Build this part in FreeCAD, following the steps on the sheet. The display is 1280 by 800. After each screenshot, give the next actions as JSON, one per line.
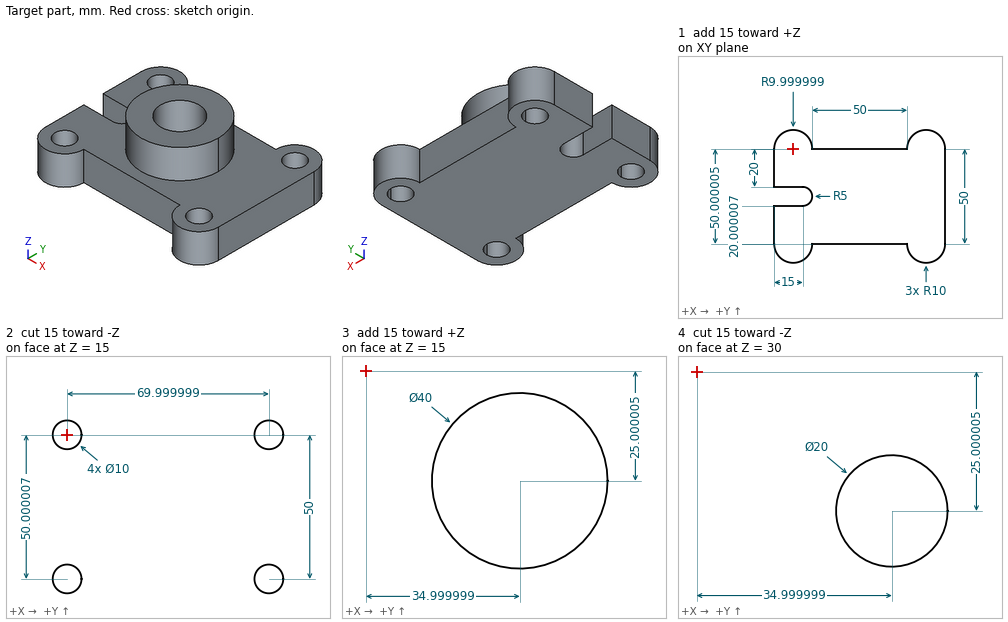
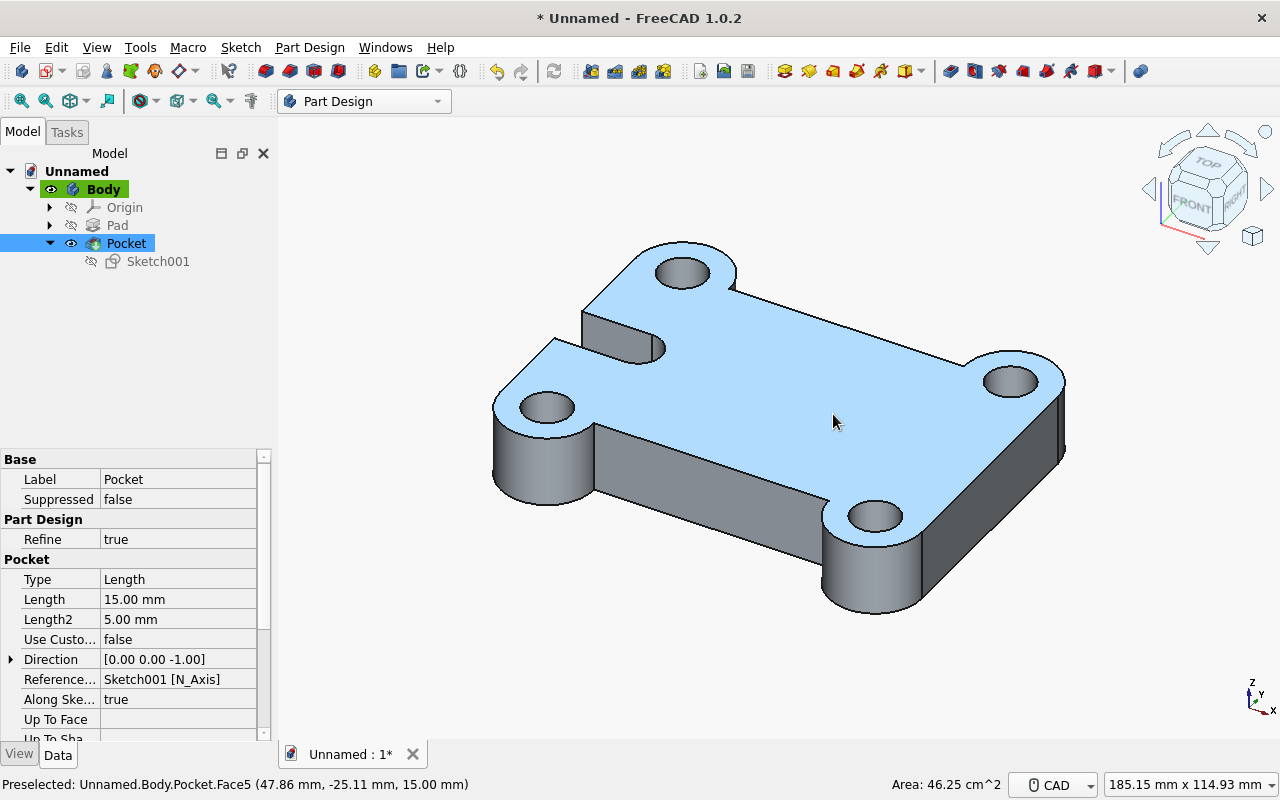
{"action": "left_click", "coordinate": [46, 72]}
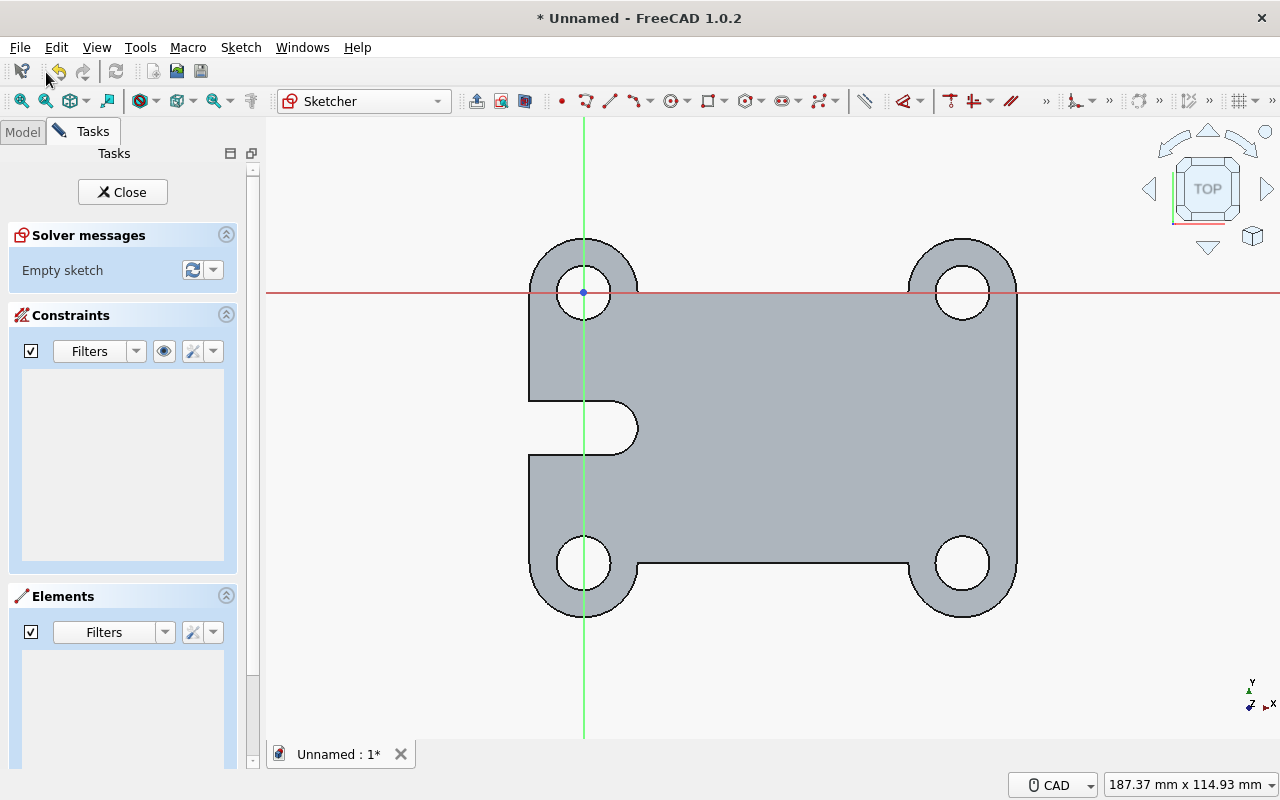
{"action": "scroll", "coordinate": [789, 387], "scroll_direction": "up", "scroll_amount": 2}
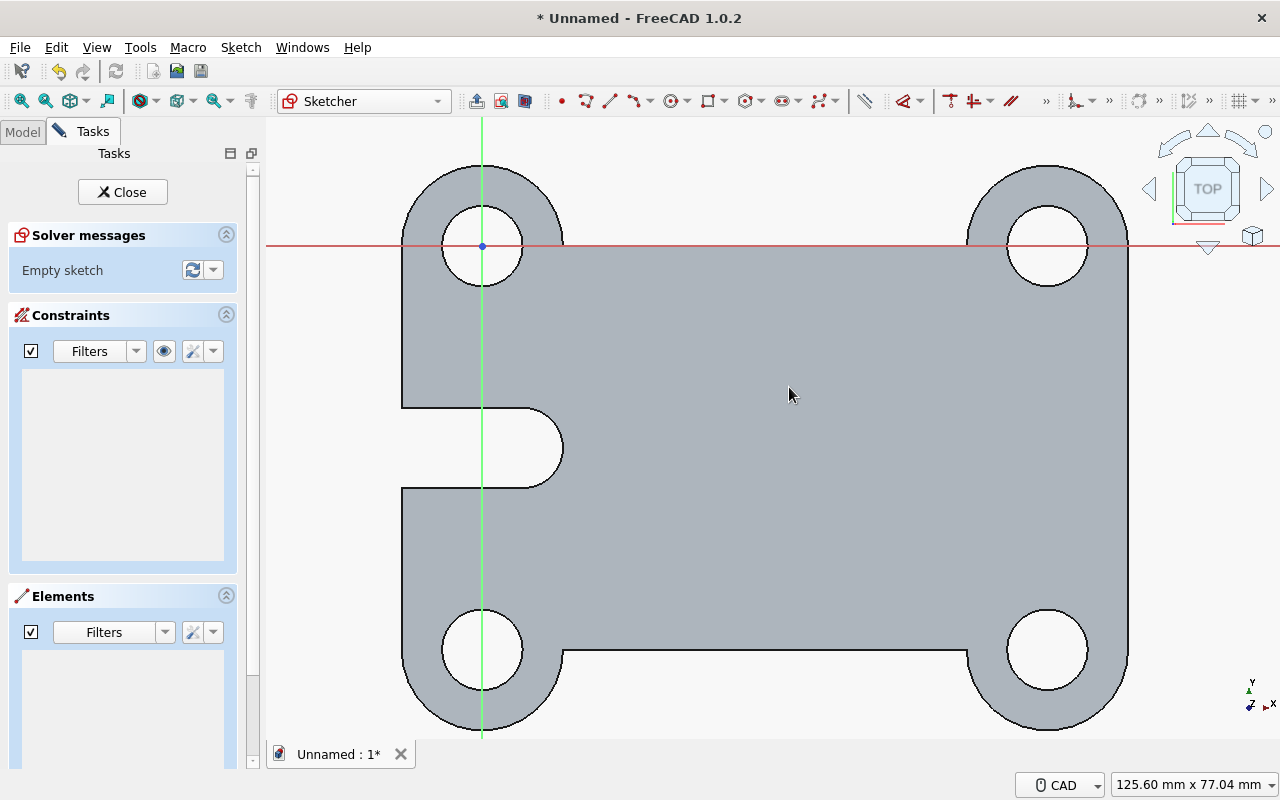
{"action": "left_click", "coordinate": [672, 102]}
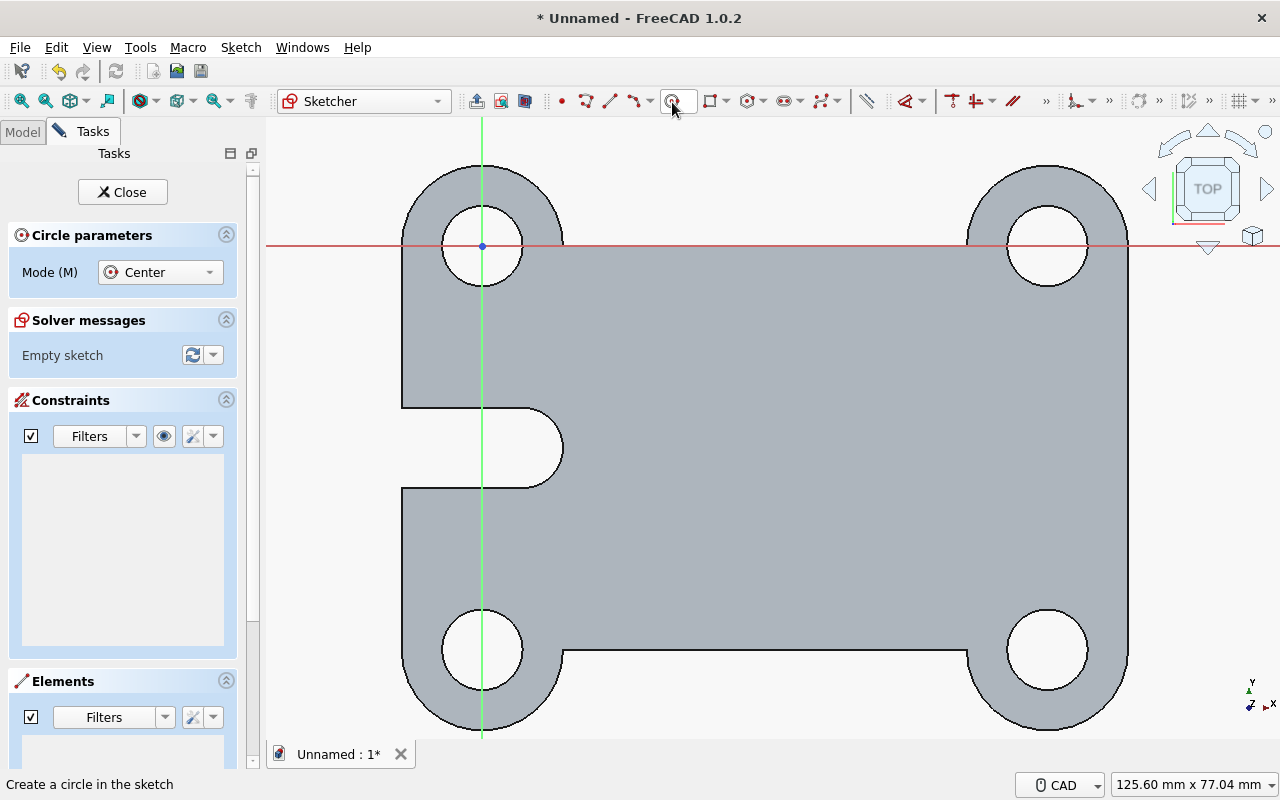
{"action": "left_click", "coordinate": [765, 448]}
{"action": "mouse_move", "coordinate": [879, 334]}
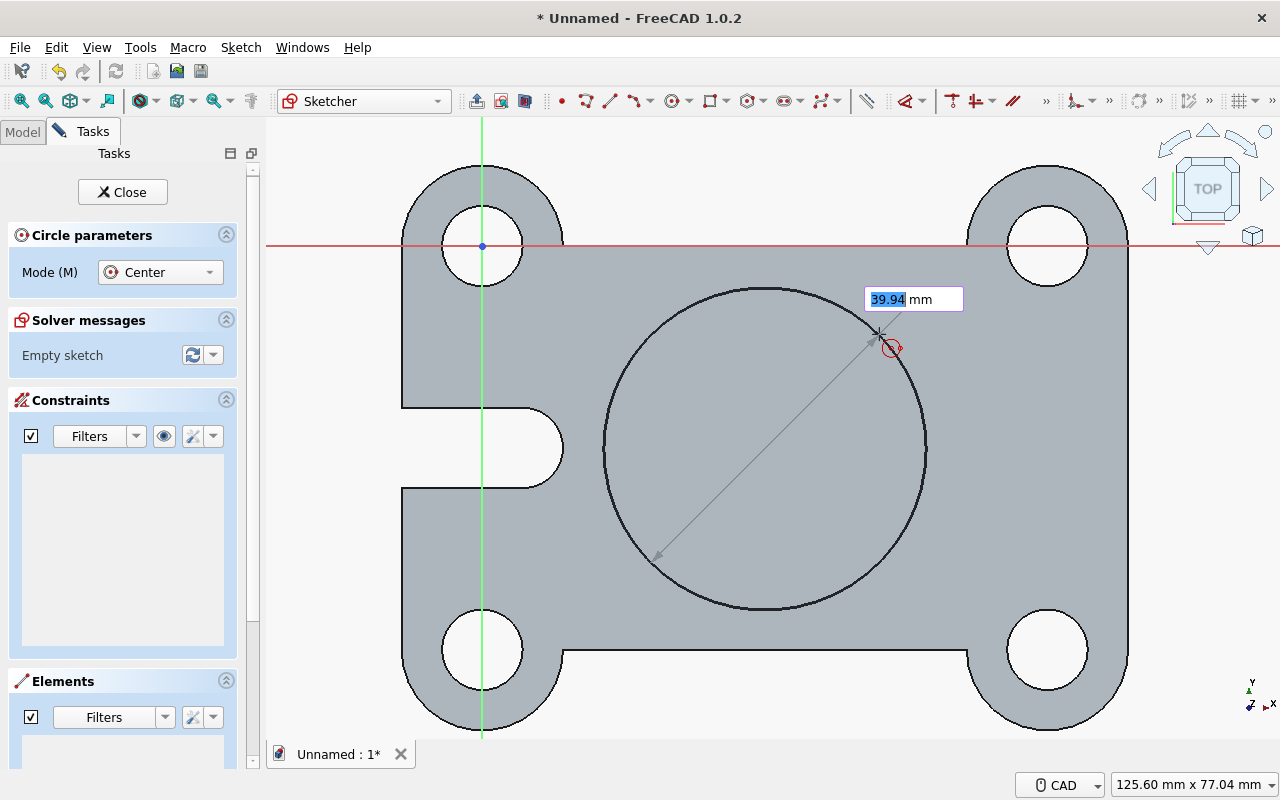
{"action": "type", "text": "40"}
{"action": "key", "text": "Return"}
{"action": "key", "text": "Escape"}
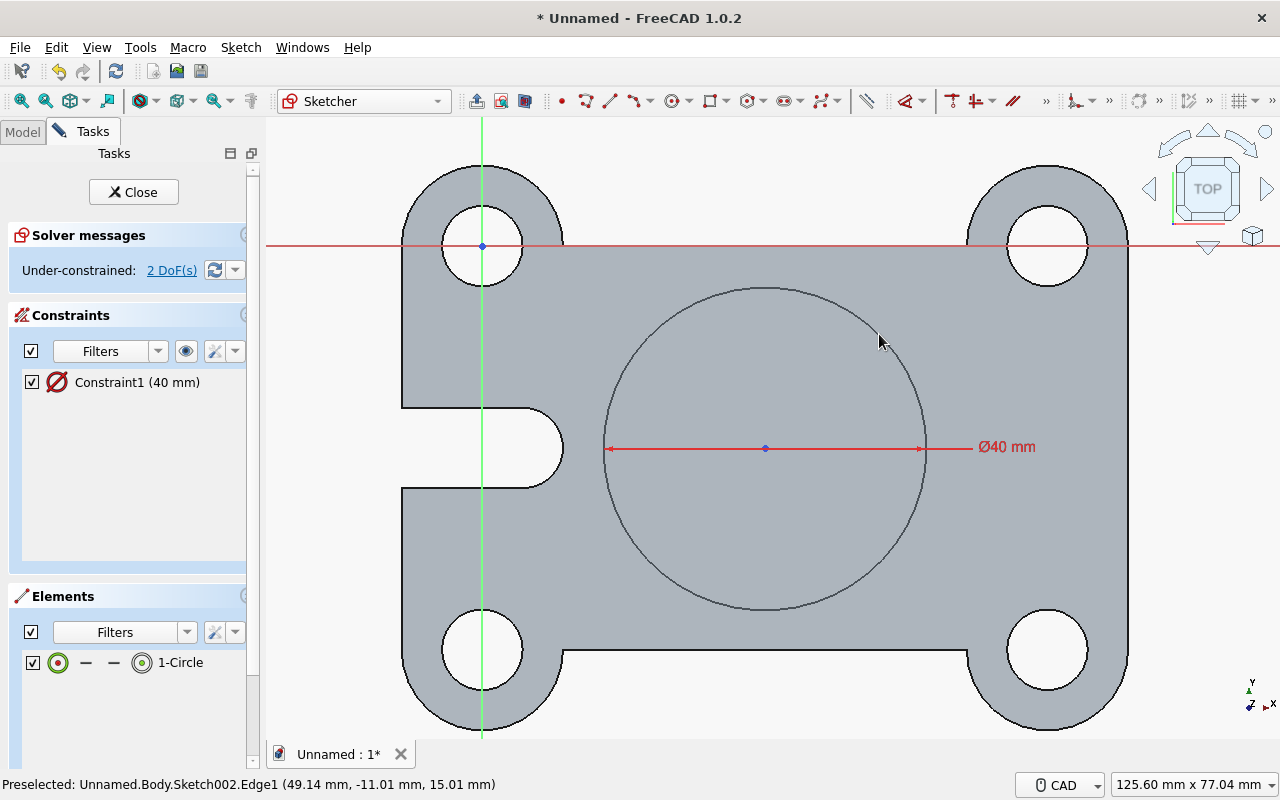
{"action": "left_click", "coordinate": [906, 102]}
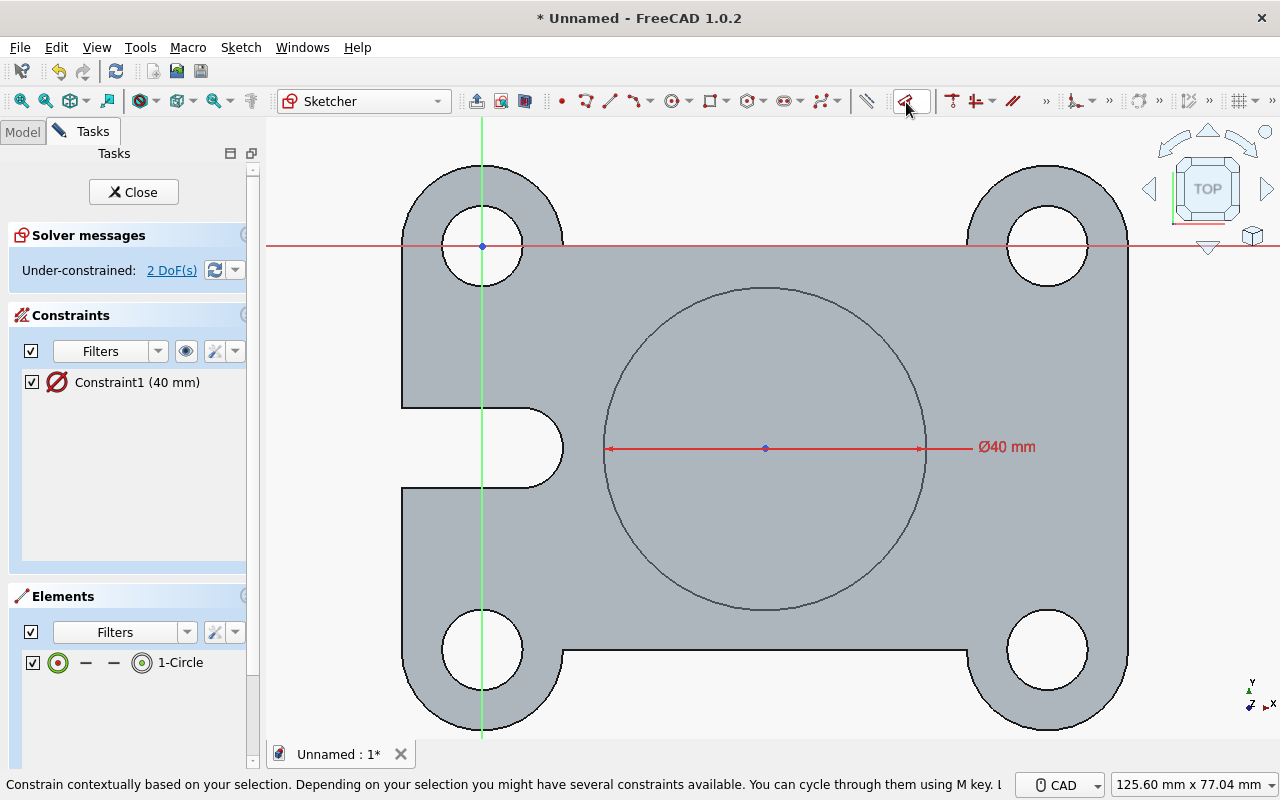
{"action": "left_click", "coordinate": [765, 449]}
{"action": "left_click", "coordinate": [624, 212]}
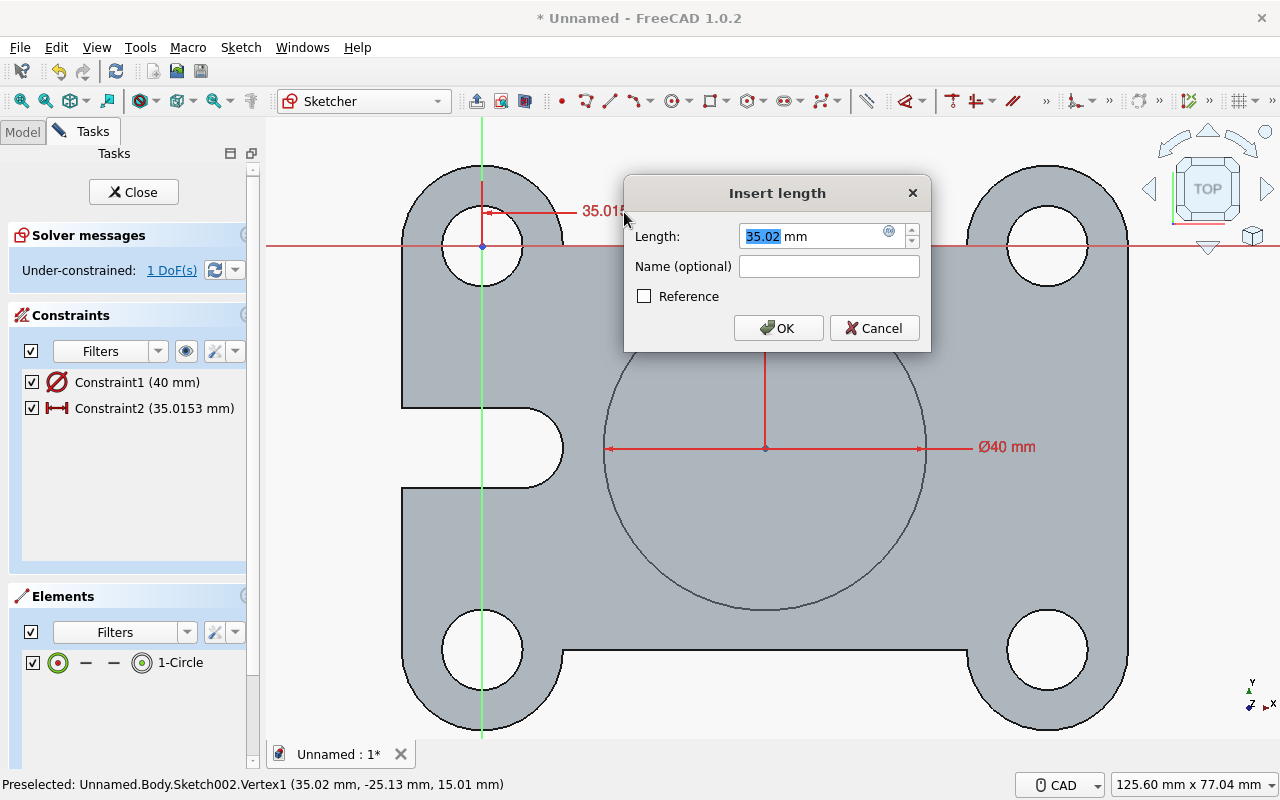
{"action": "type", "text": "34.999999"}
{"action": "key", "text": "Return"}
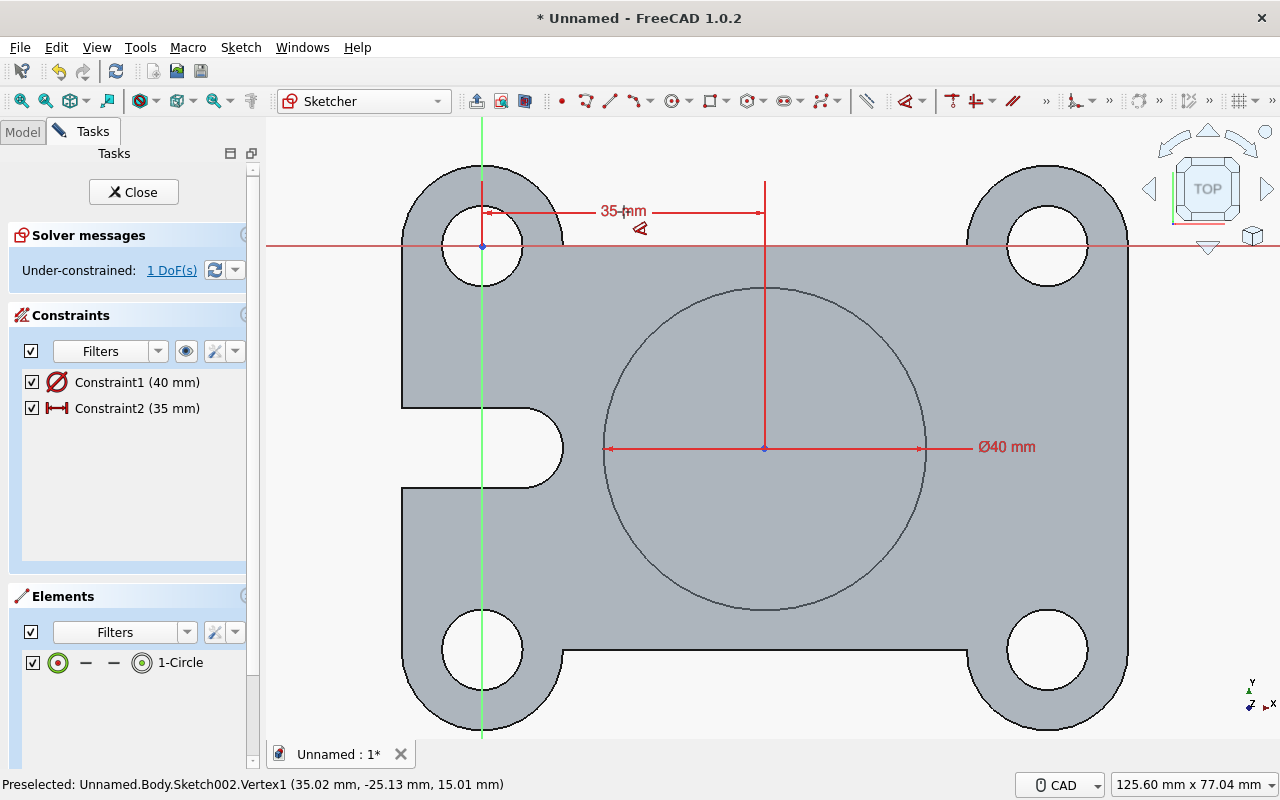
{"action": "left_click", "coordinate": [765, 449]}
{"action": "left_click", "coordinate": [448, 348]}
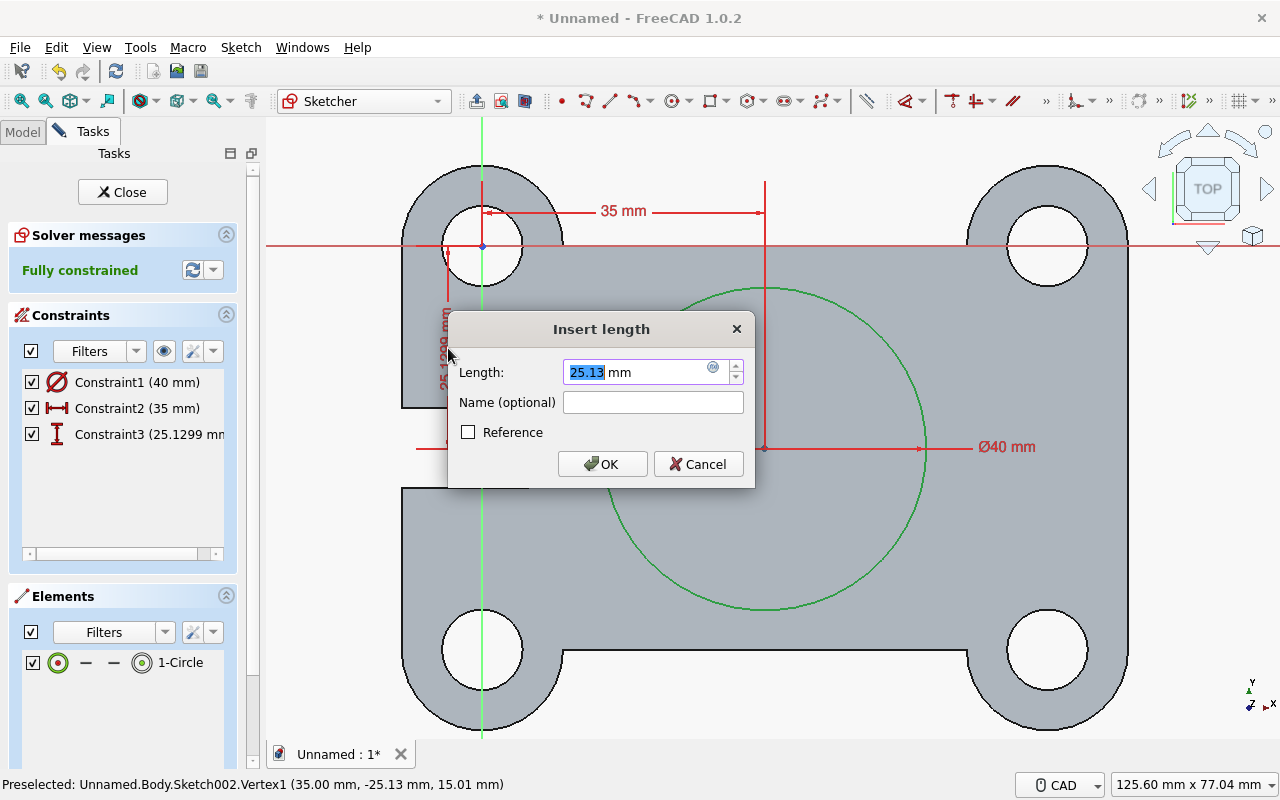
{"action": "type", "text": "25.000005"}
{"action": "key", "text": "Return"}
{"action": "key", "text": "Escape"}